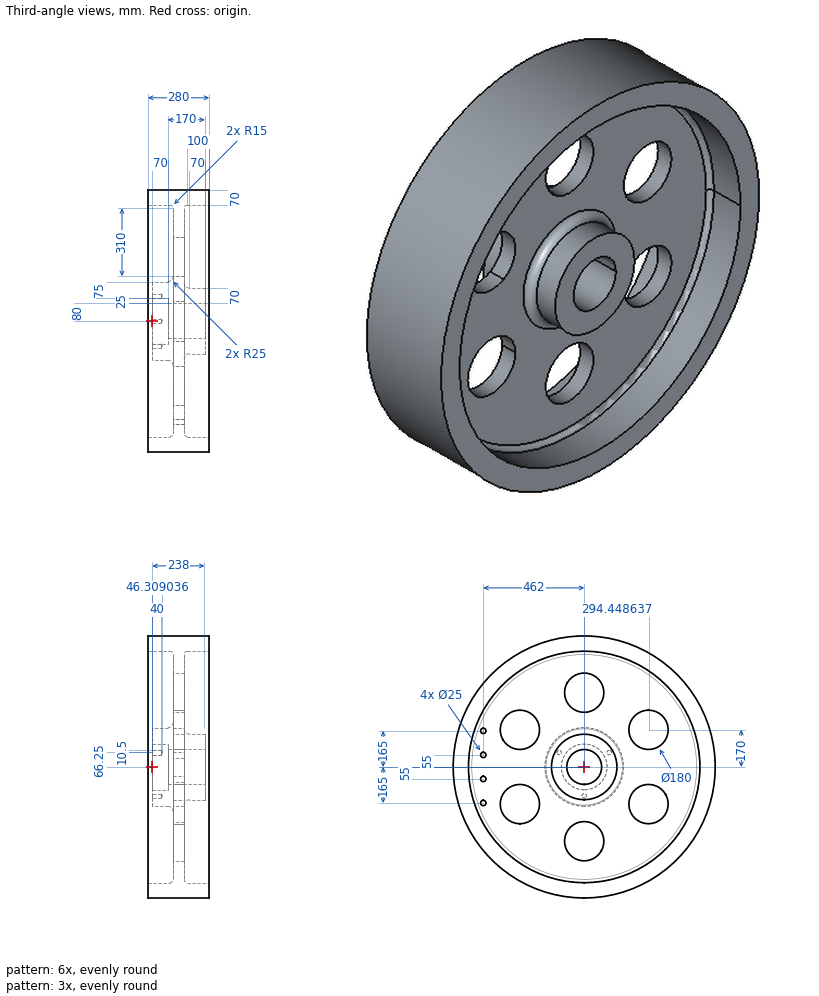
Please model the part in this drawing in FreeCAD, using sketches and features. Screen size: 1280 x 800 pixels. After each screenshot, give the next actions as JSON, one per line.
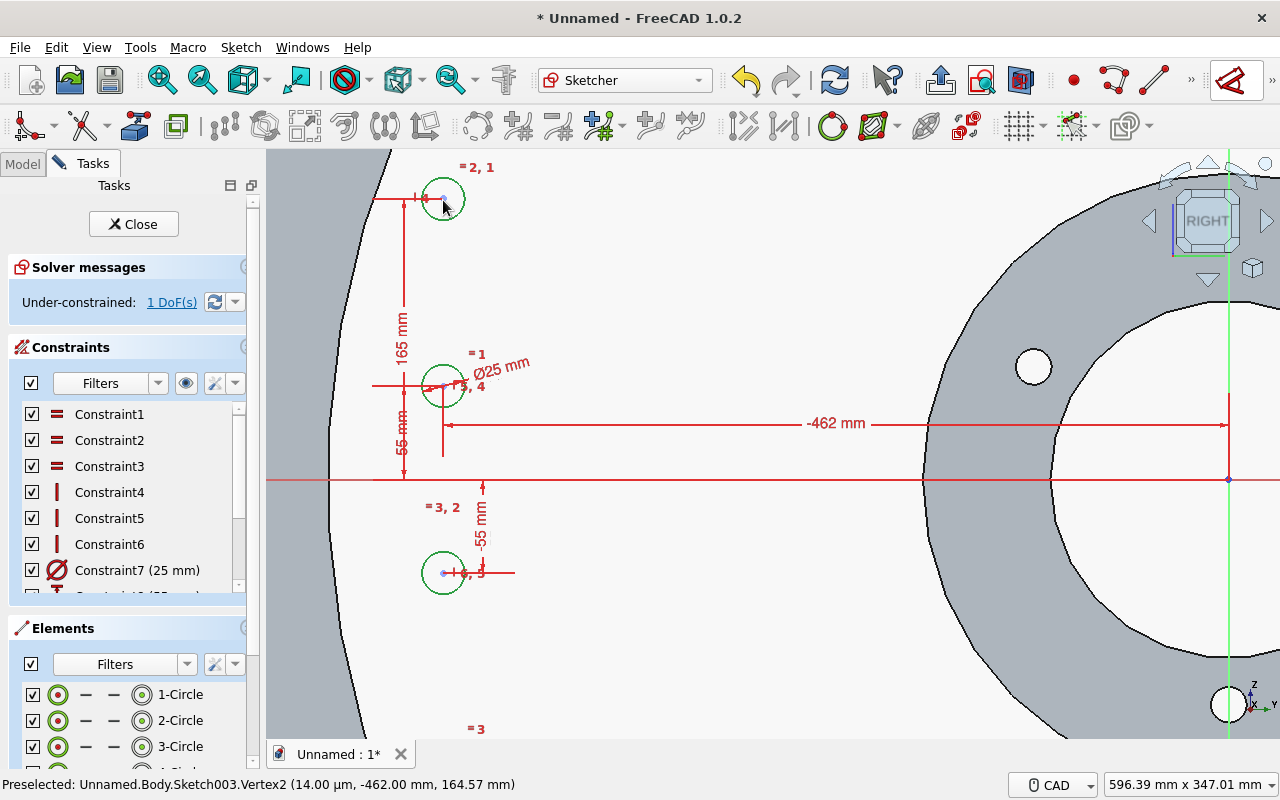
{"action": "scroll", "coordinate": [458, 372], "scroll_direction": "down", "scroll_amount": 2}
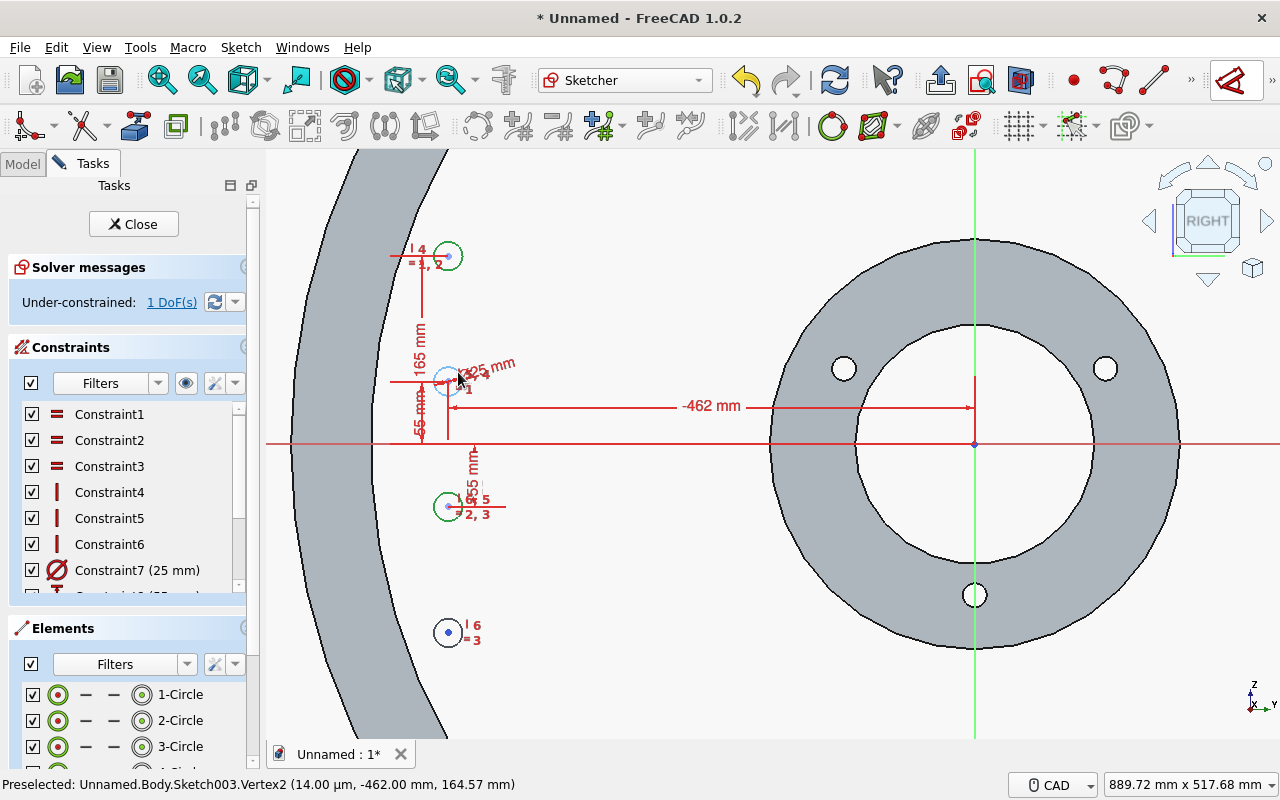
{"action": "left_click", "coordinate": [448, 633]}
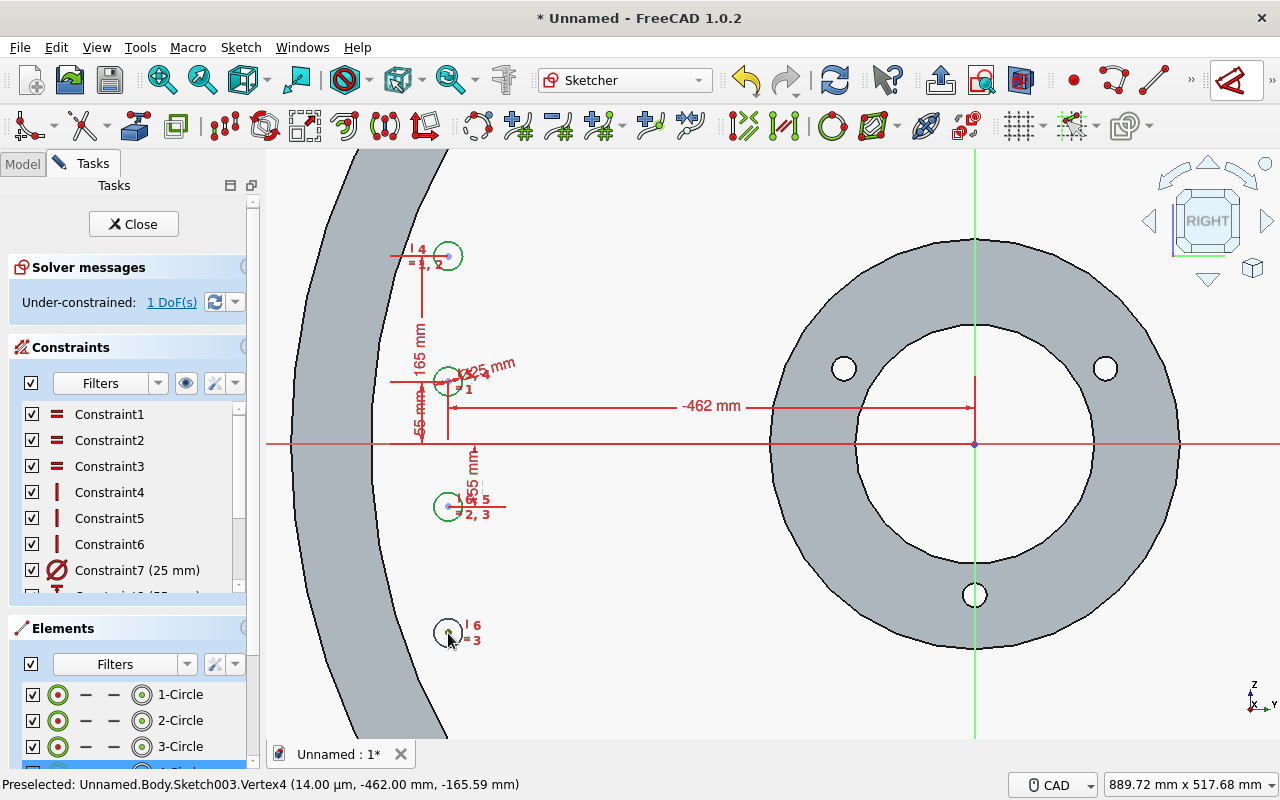
{"action": "left_click", "coordinate": [1258, 80]}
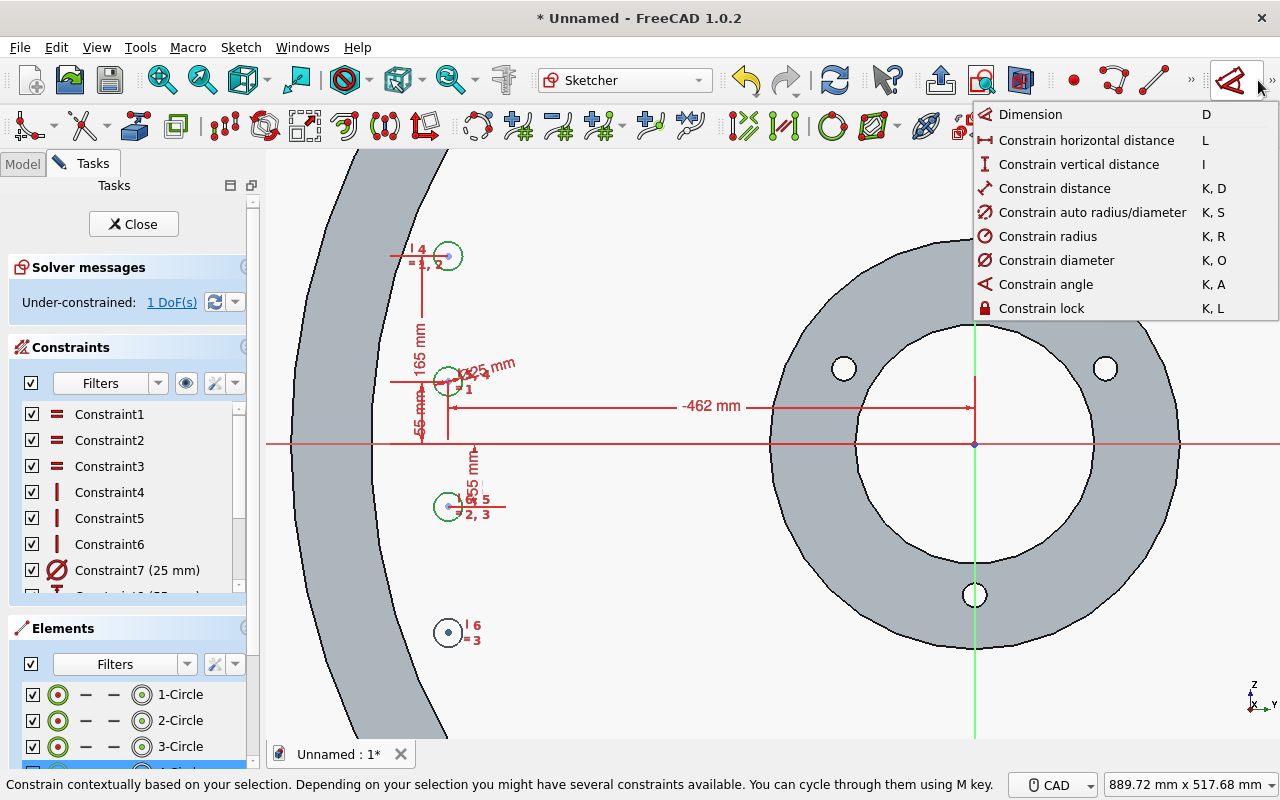
{"action": "left_click", "coordinate": [1126, 164]}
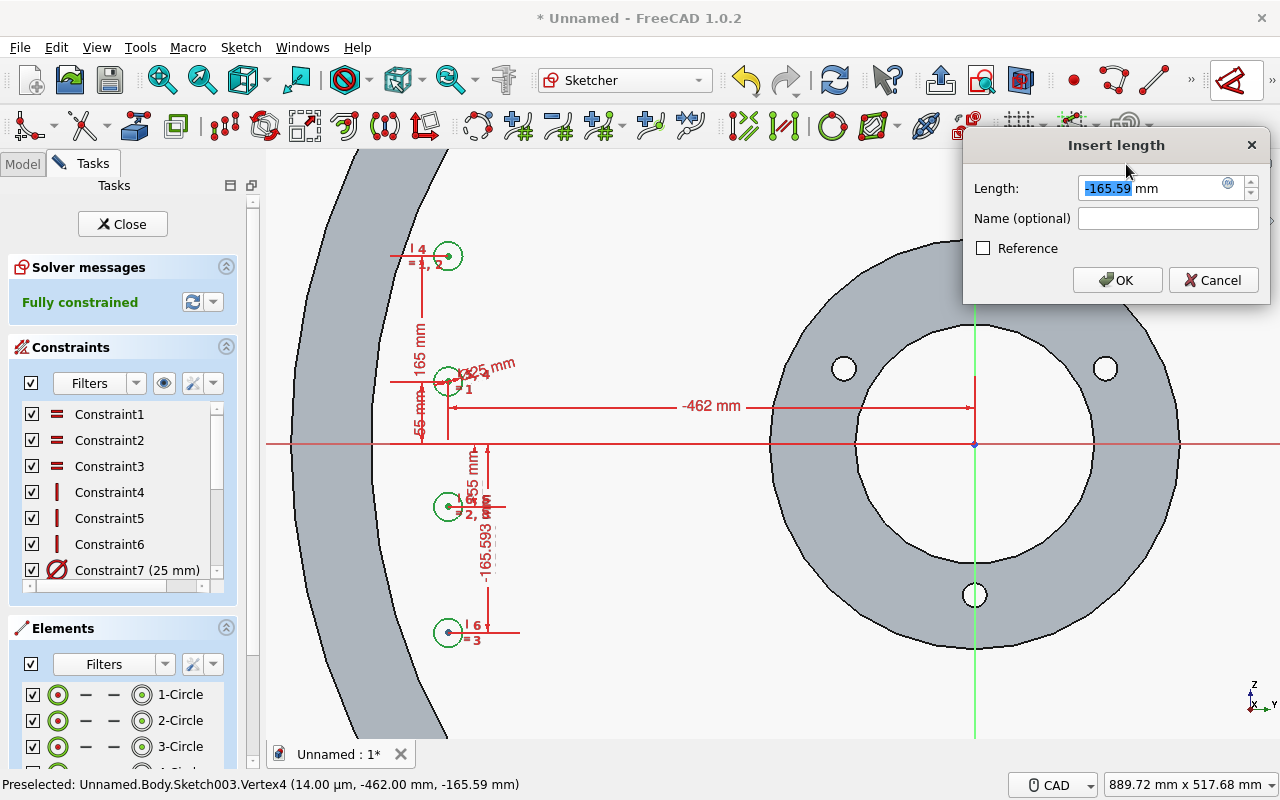
{"action": "type", "text": "-165"}
{"action": "key", "text": "Return"}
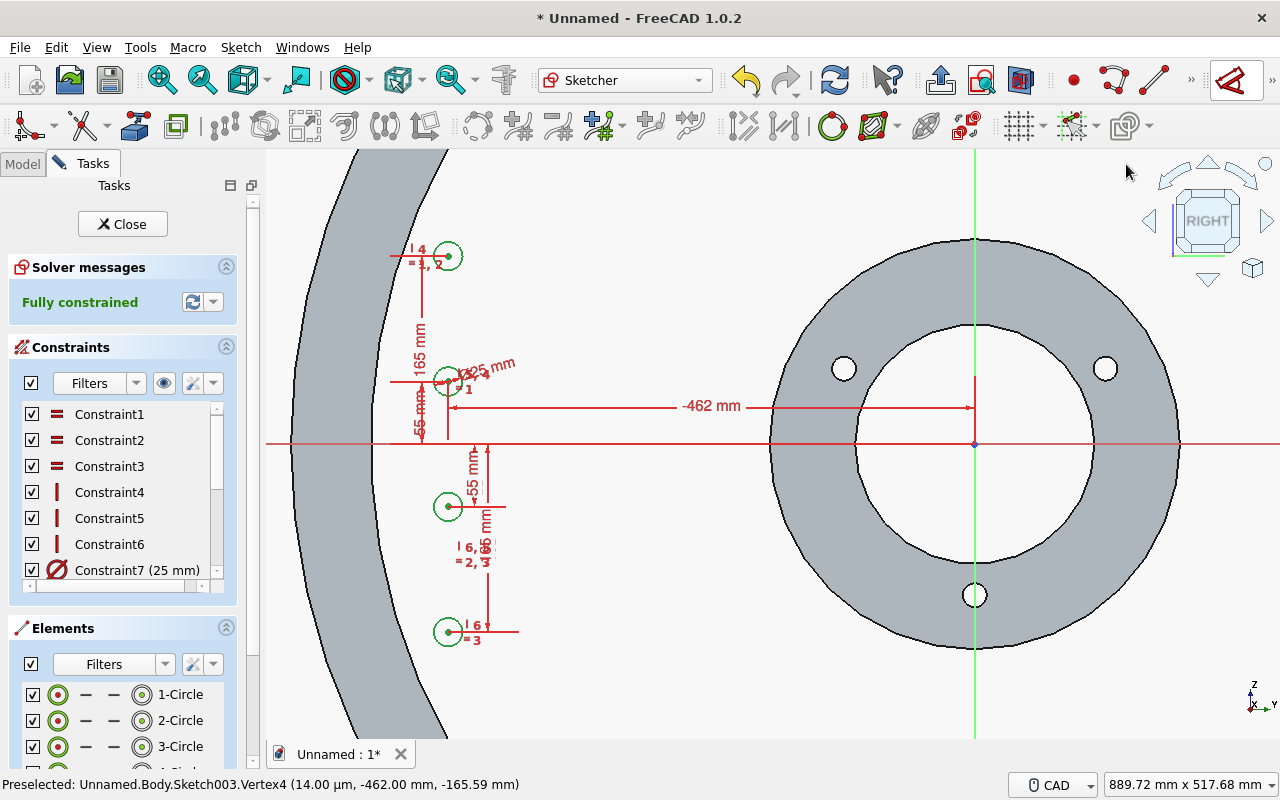
{"action": "left_click", "coordinate": [123, 224]}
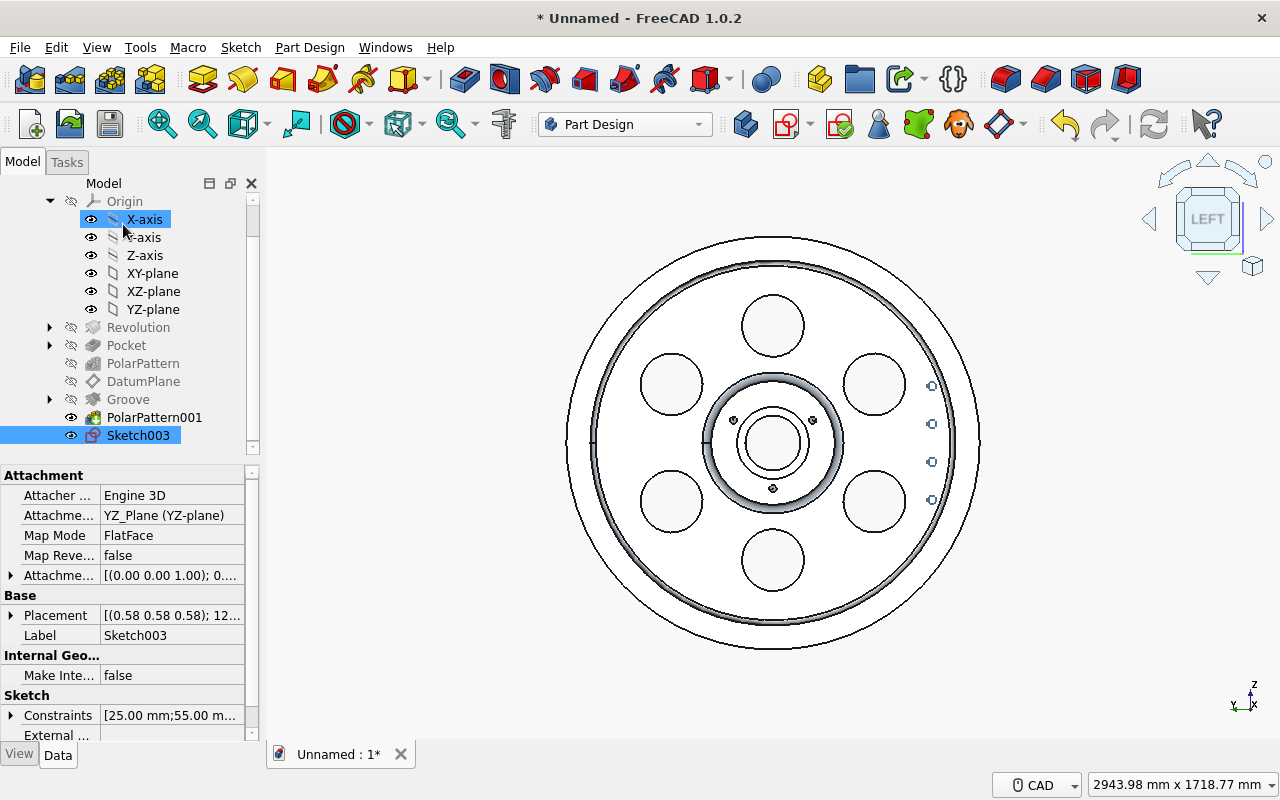
{"action": "left_click", "coordinate": [466, 80]}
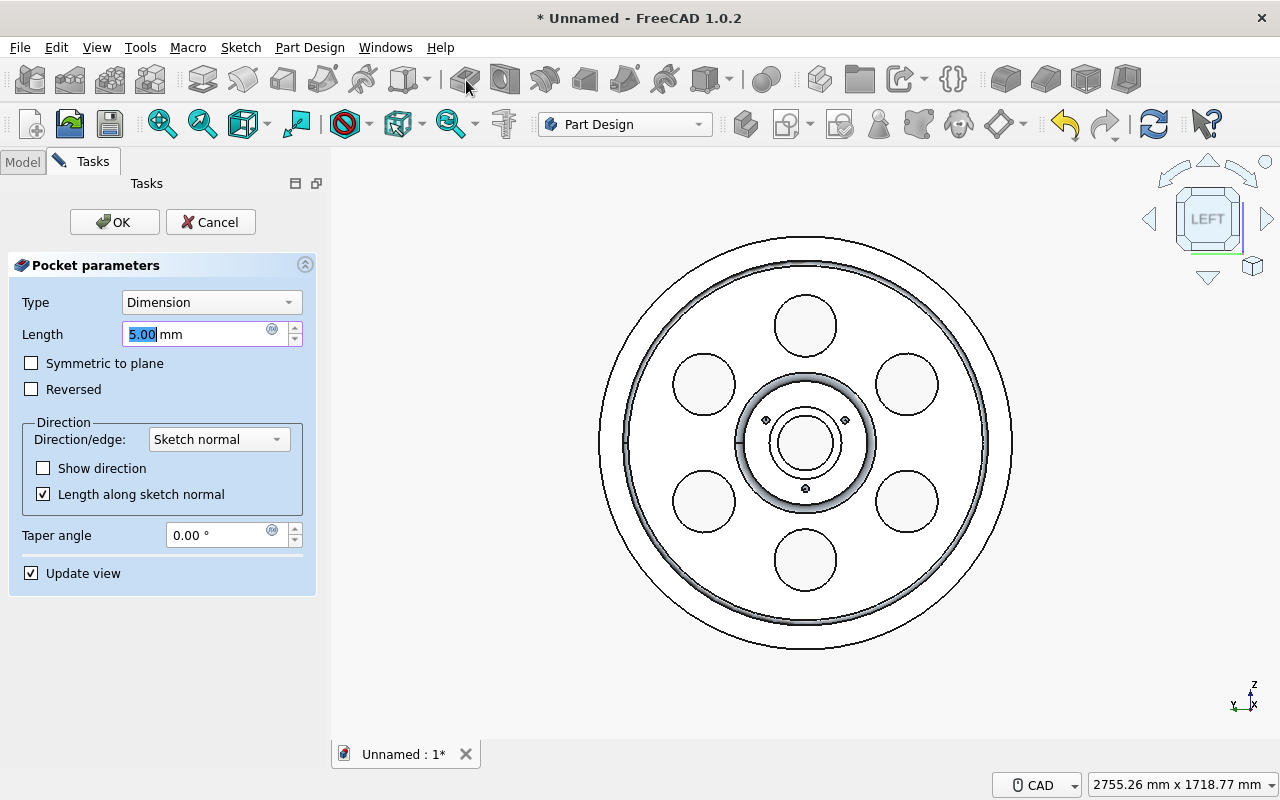
{"action": "type", "text": "238"}
{"action": "key", "text": "Tab"}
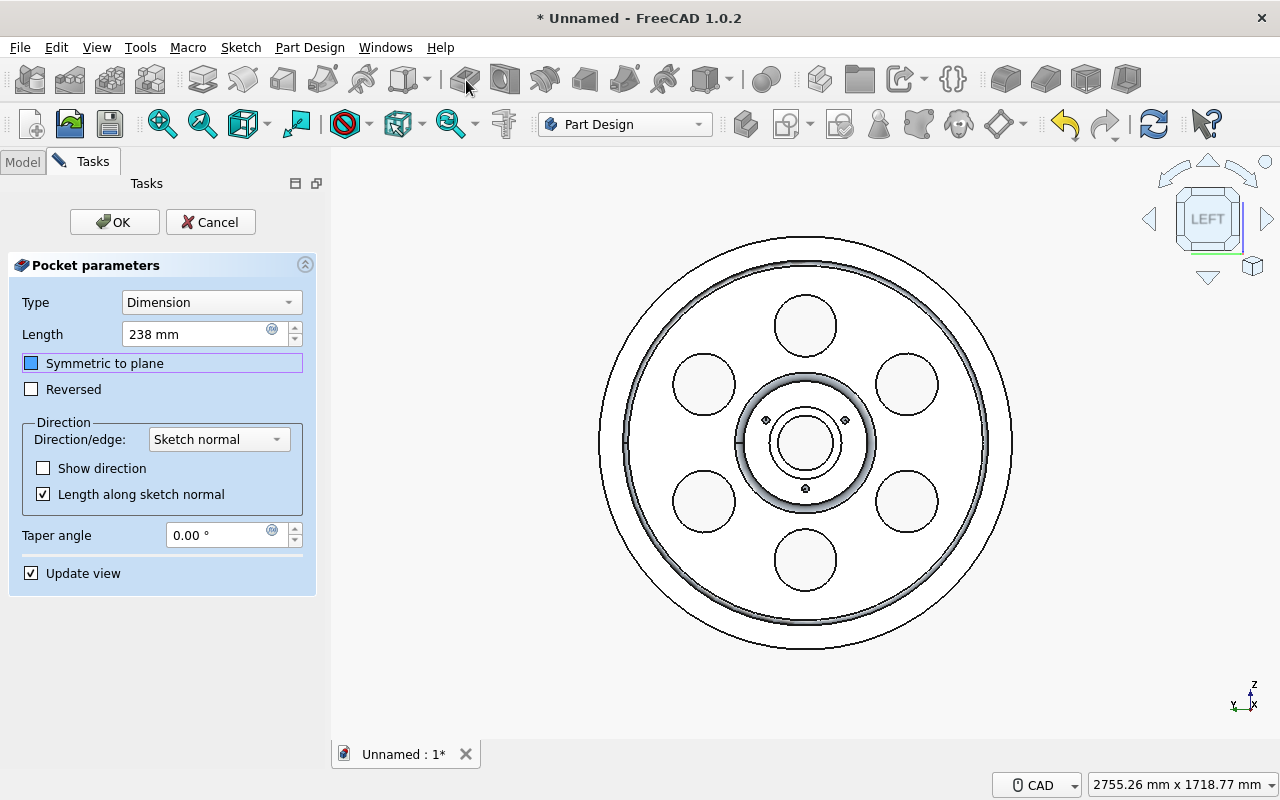
{"action": "left_click", "coordinate": [30, 389]}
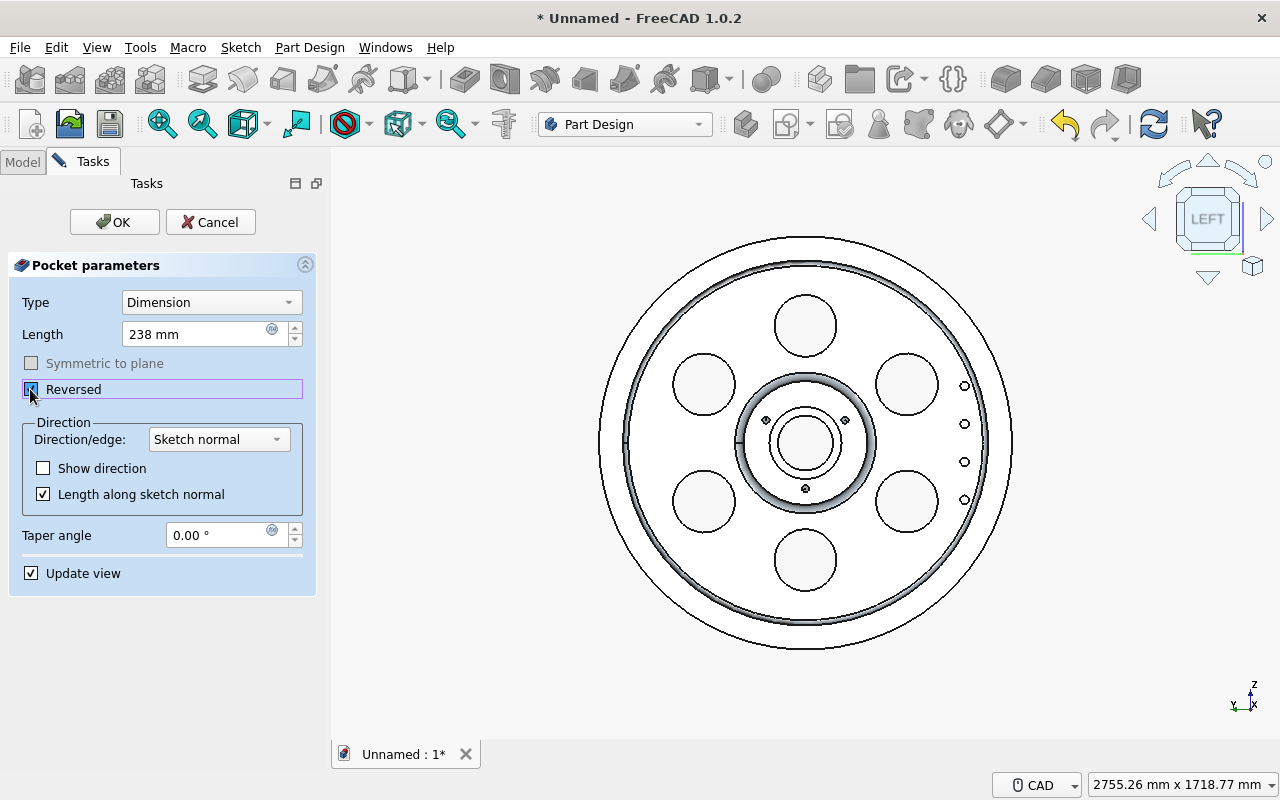
{"action": "left_click", "coordinate": [115, 222]}